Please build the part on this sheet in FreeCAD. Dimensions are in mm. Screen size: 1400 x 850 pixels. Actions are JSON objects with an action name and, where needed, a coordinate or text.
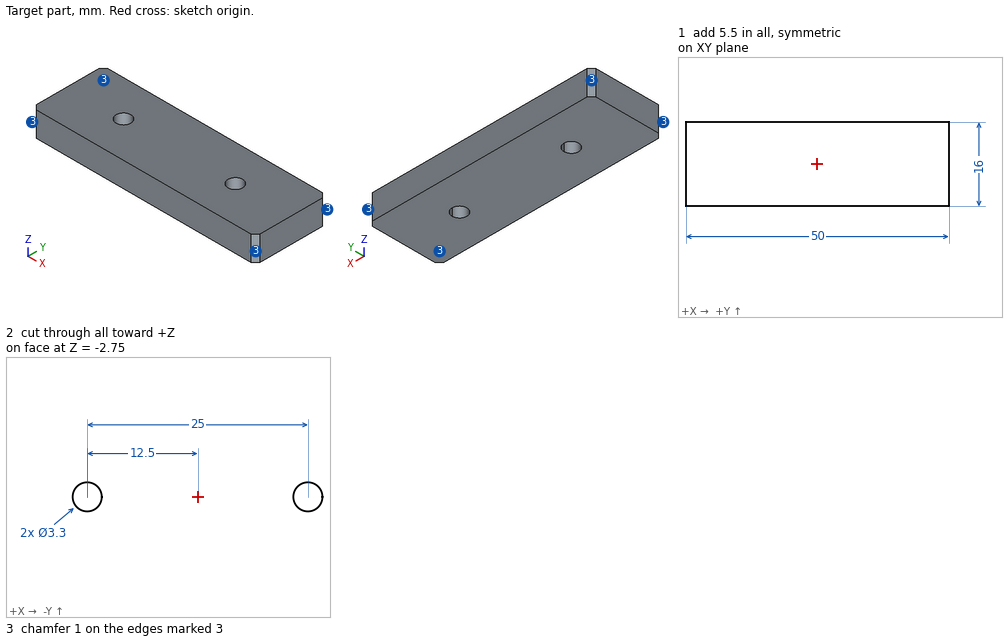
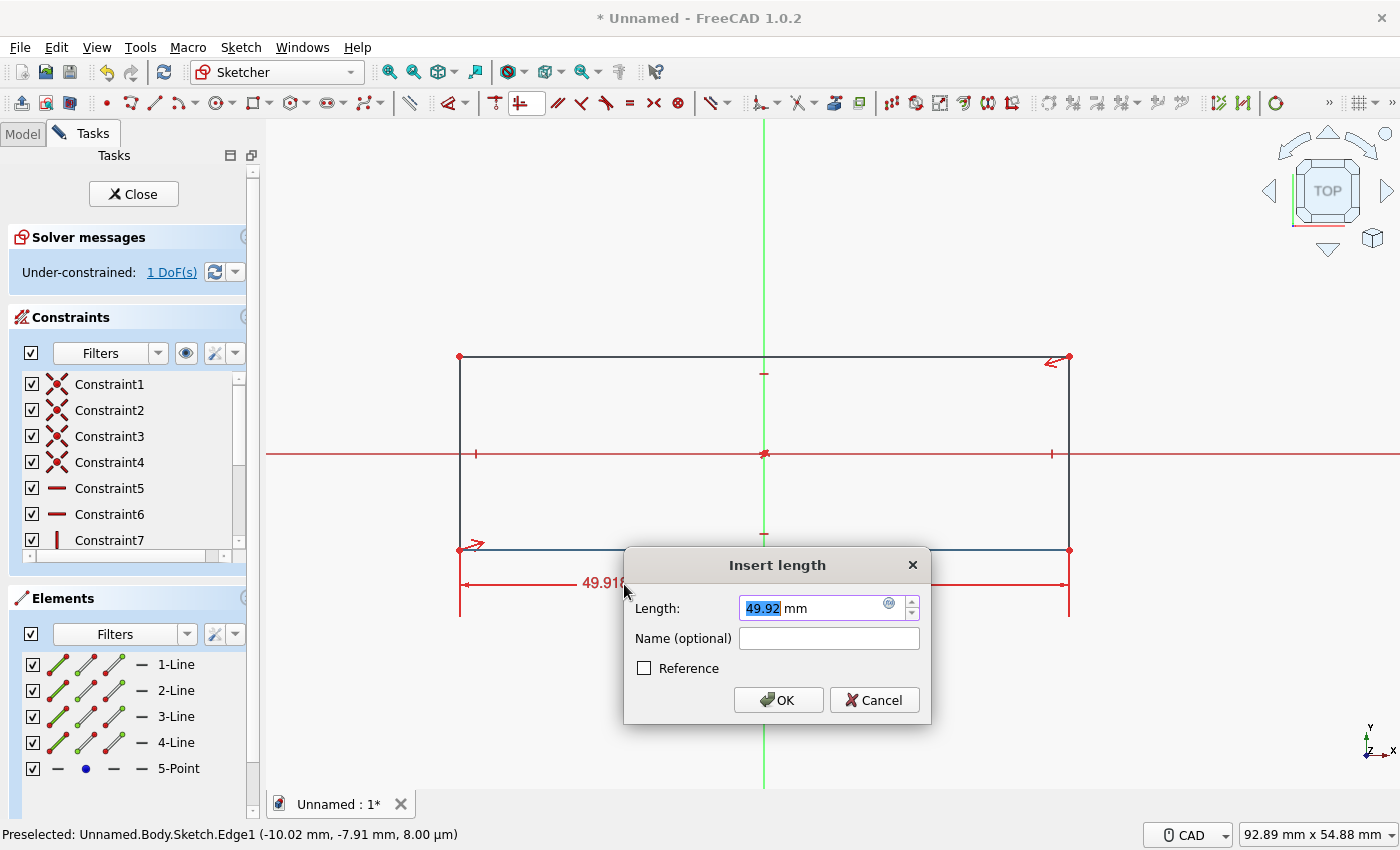
{"action": "type", "text": "50"}
{"action": "key", "text": "Return"}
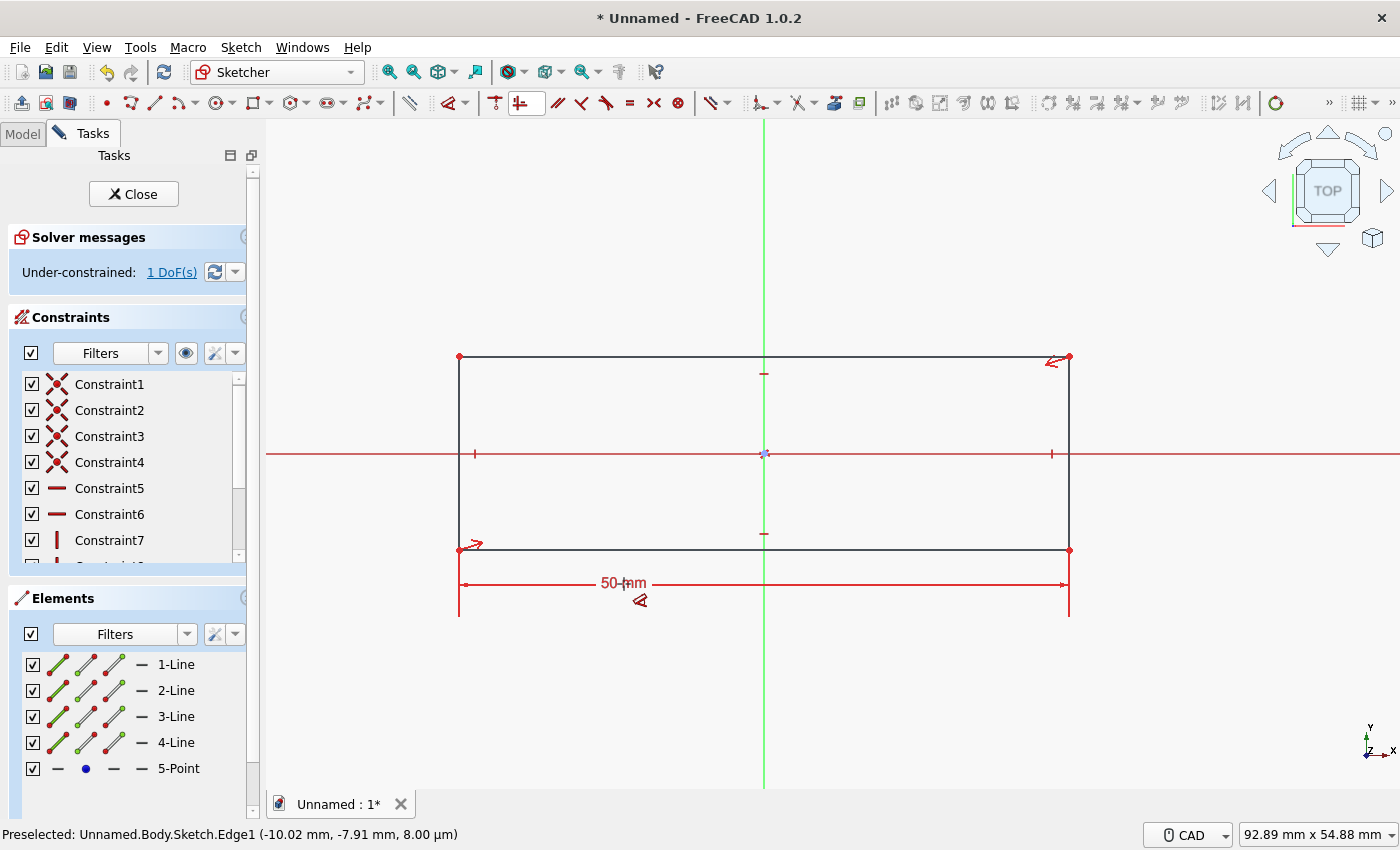
{"action": "left_click", "coordinate": [1069, 492]}
{"action": "left_click", "coordinate": [1103, 409]}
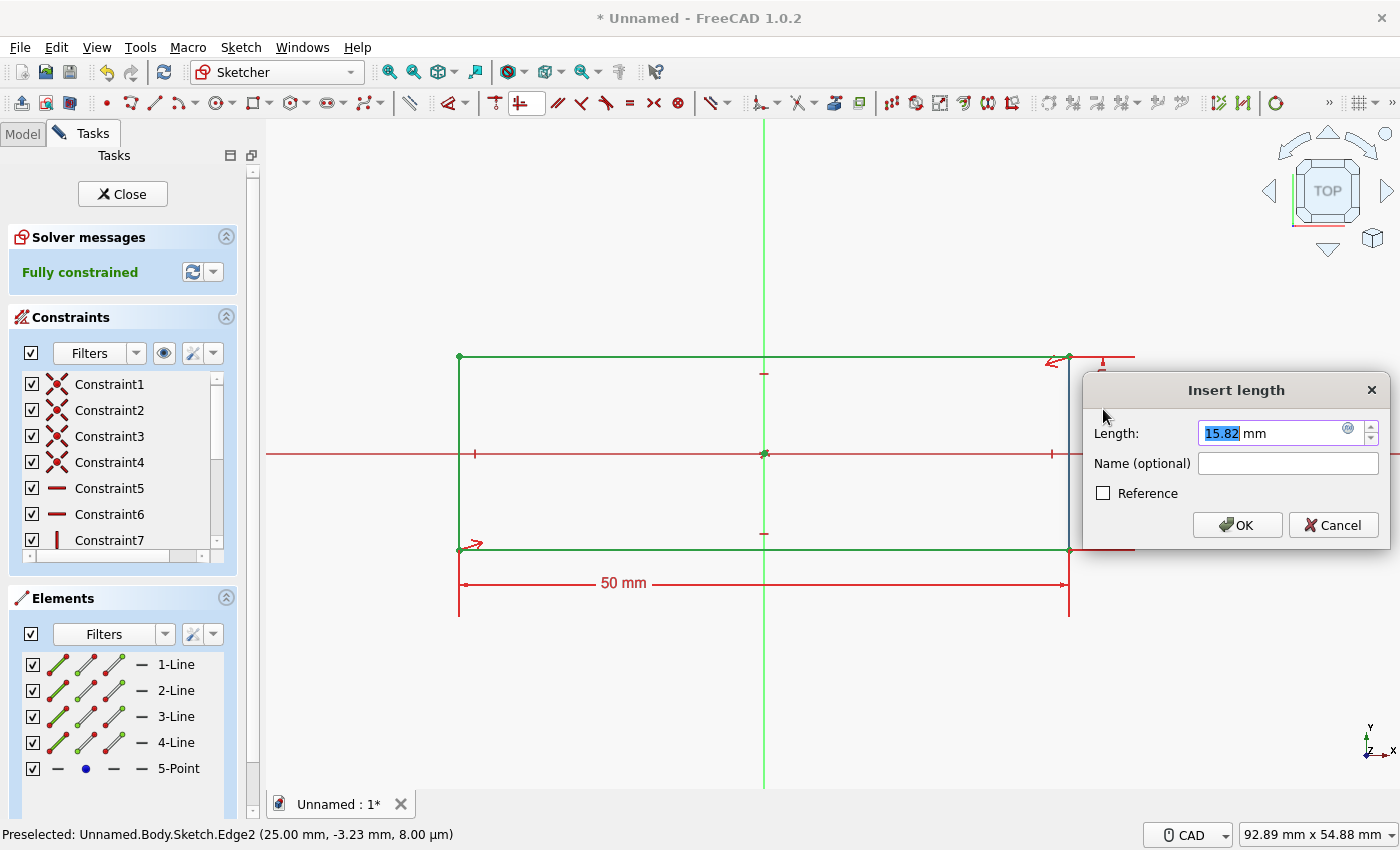
{"action": "type", "text": "16"}
{"action": "key", "text": "Return"}
{"action": "key", "text": "Escape"}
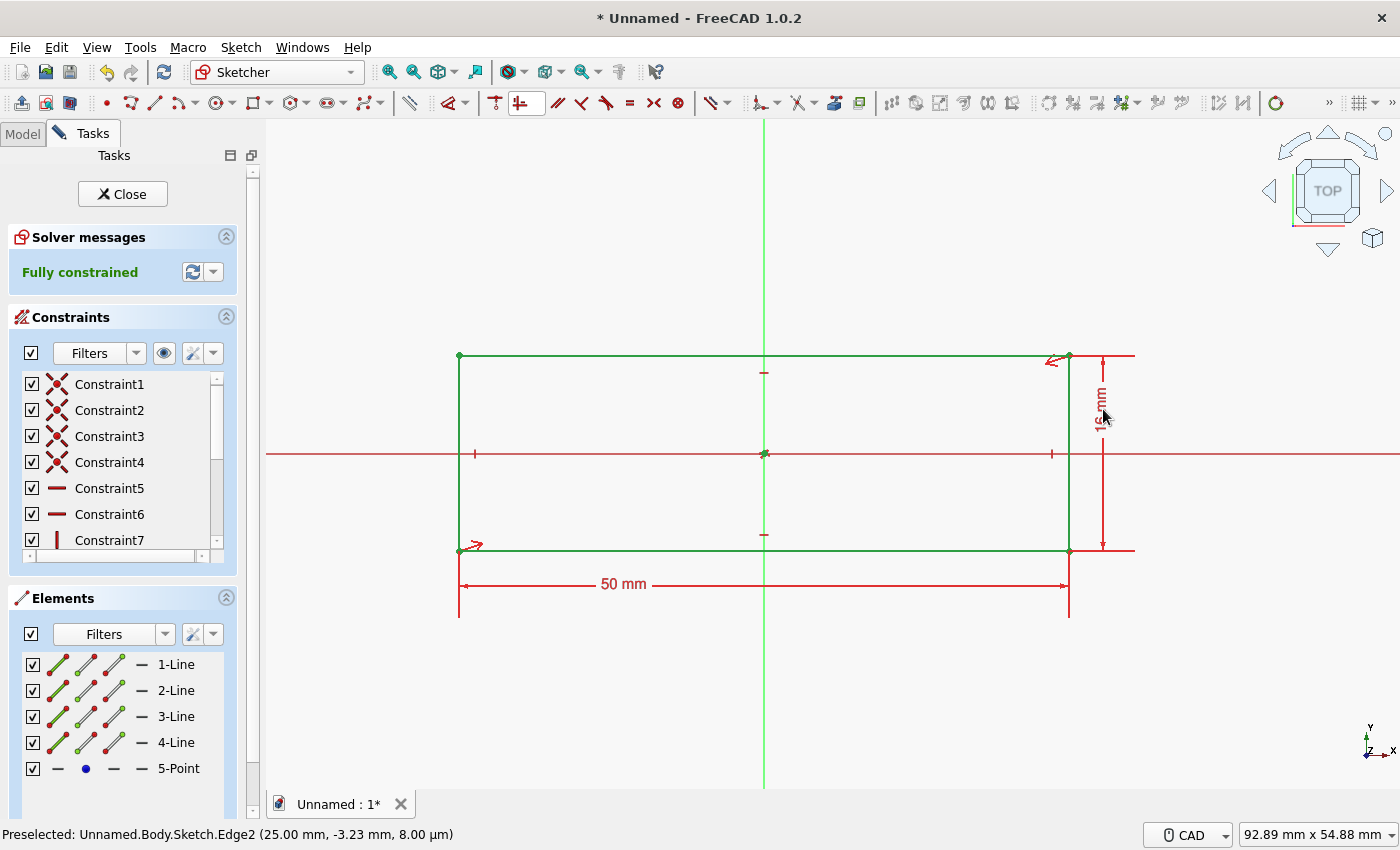
{"action": "left_click", "coordinate": [123, 194]}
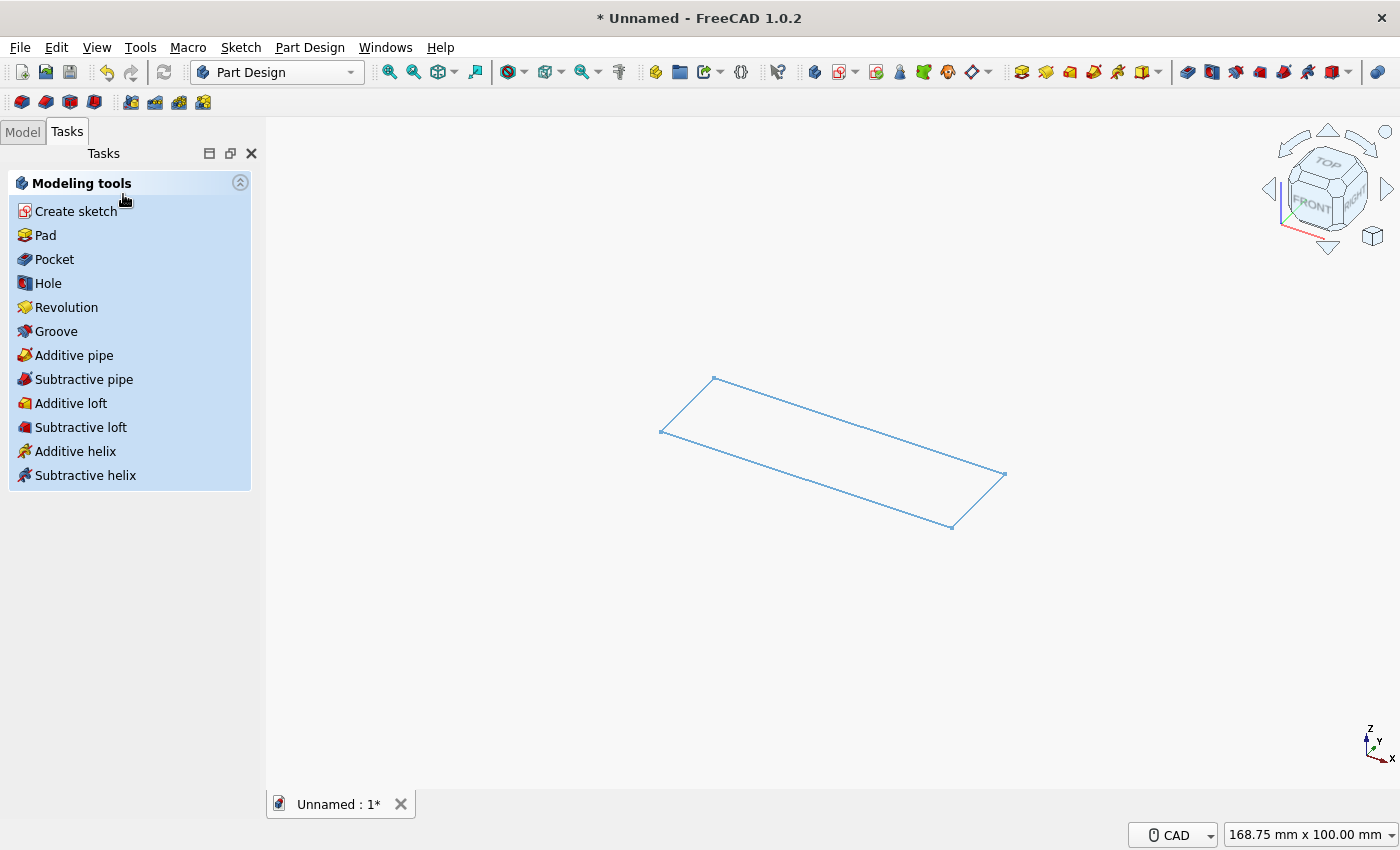
{"action": "left_click", "coordinate": [1022, 72]}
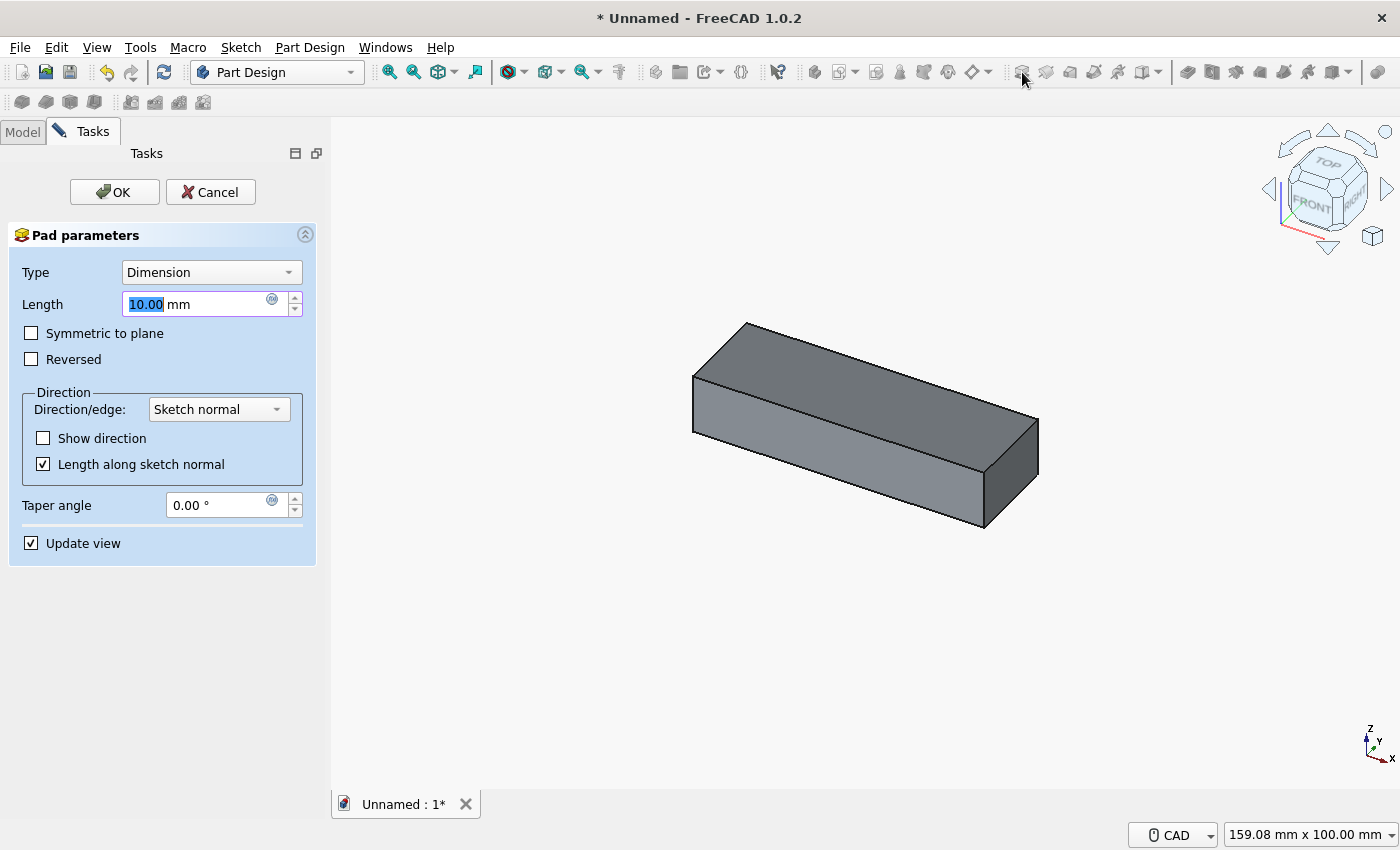
{"action": "type", "text": "5.5"}
{"action": "key", "text": "Tab"}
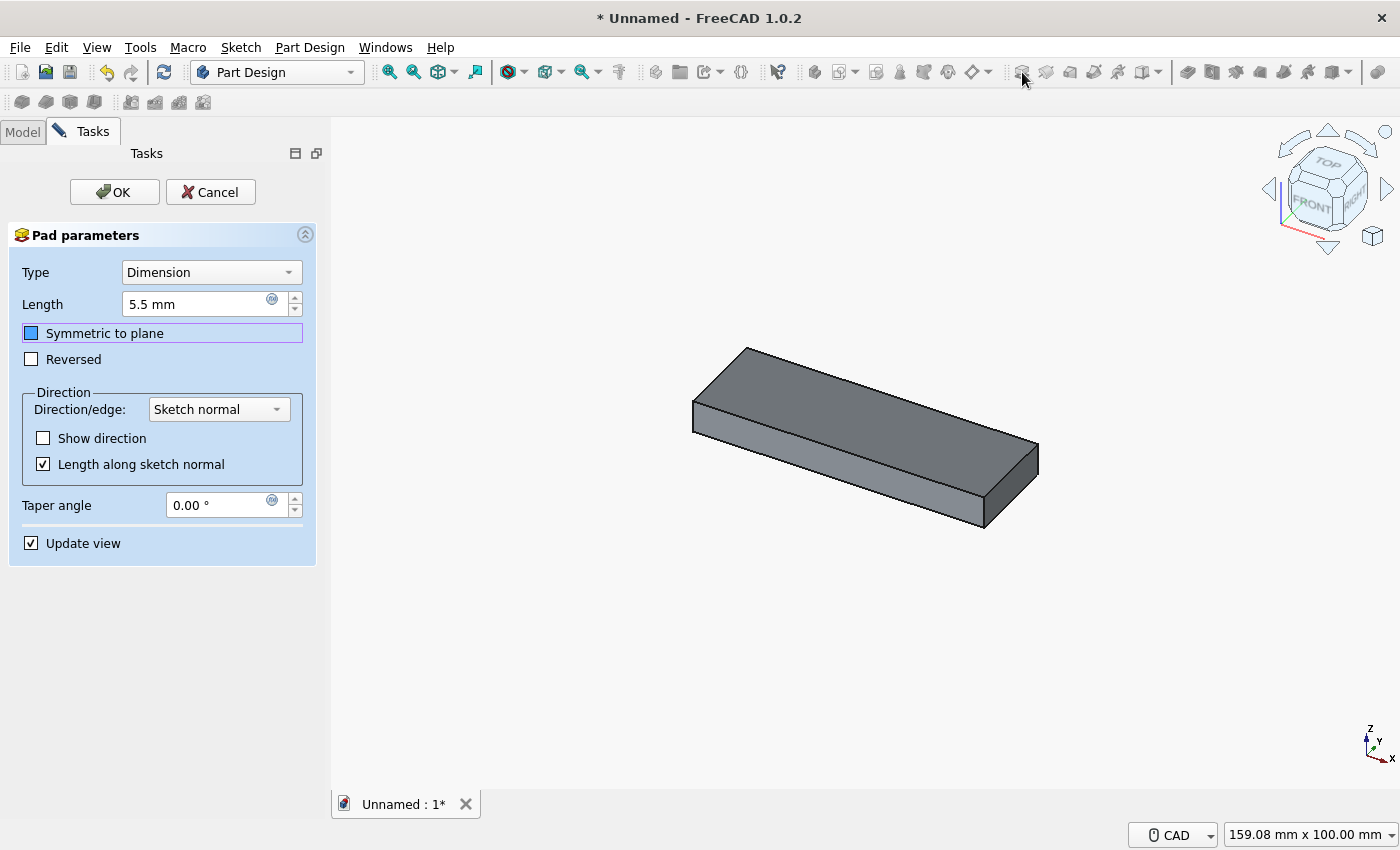
{"action": "left_click", "coordinate": [30, 333]}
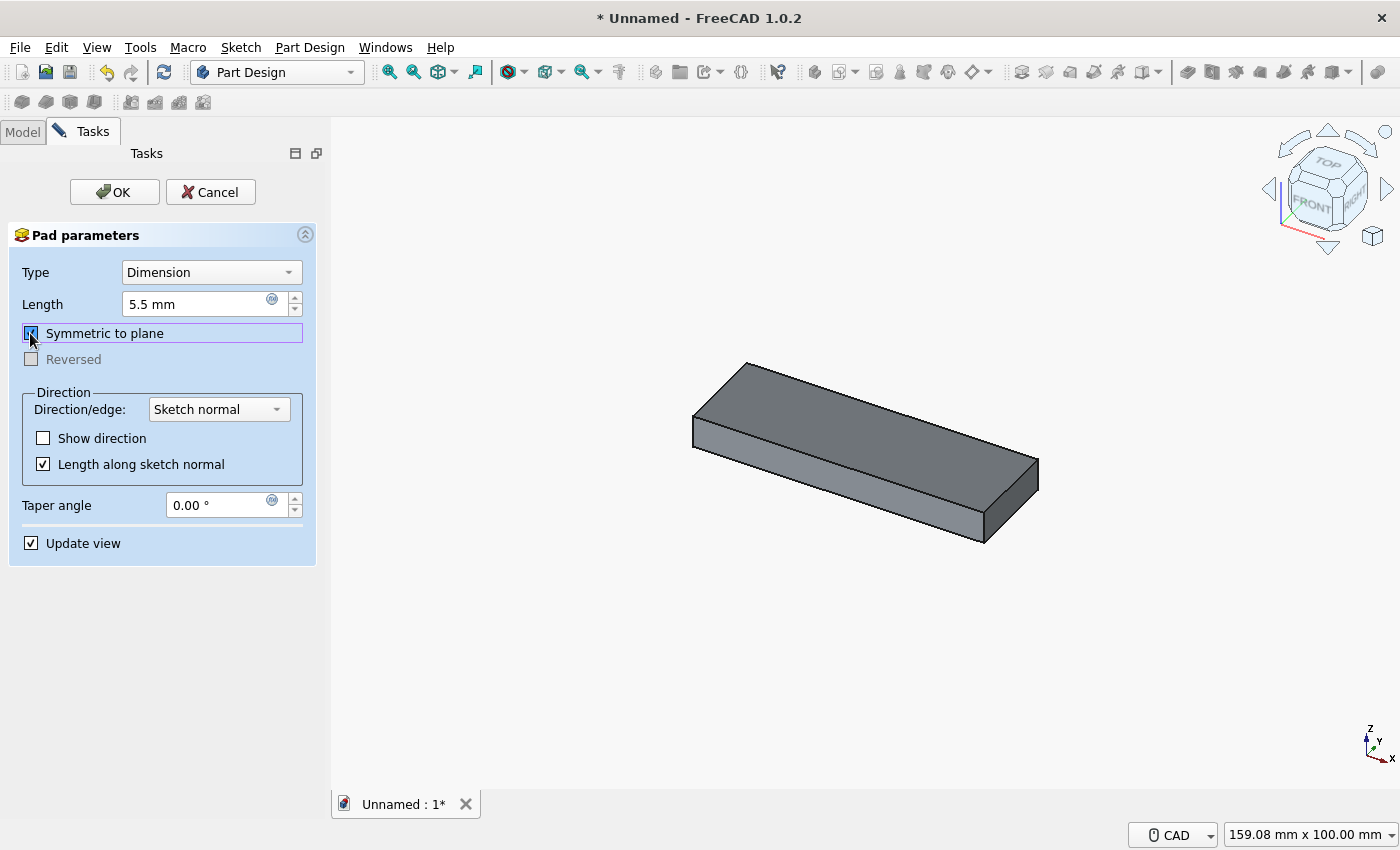
{"action": "left_click", "coordinate": [115, 192]}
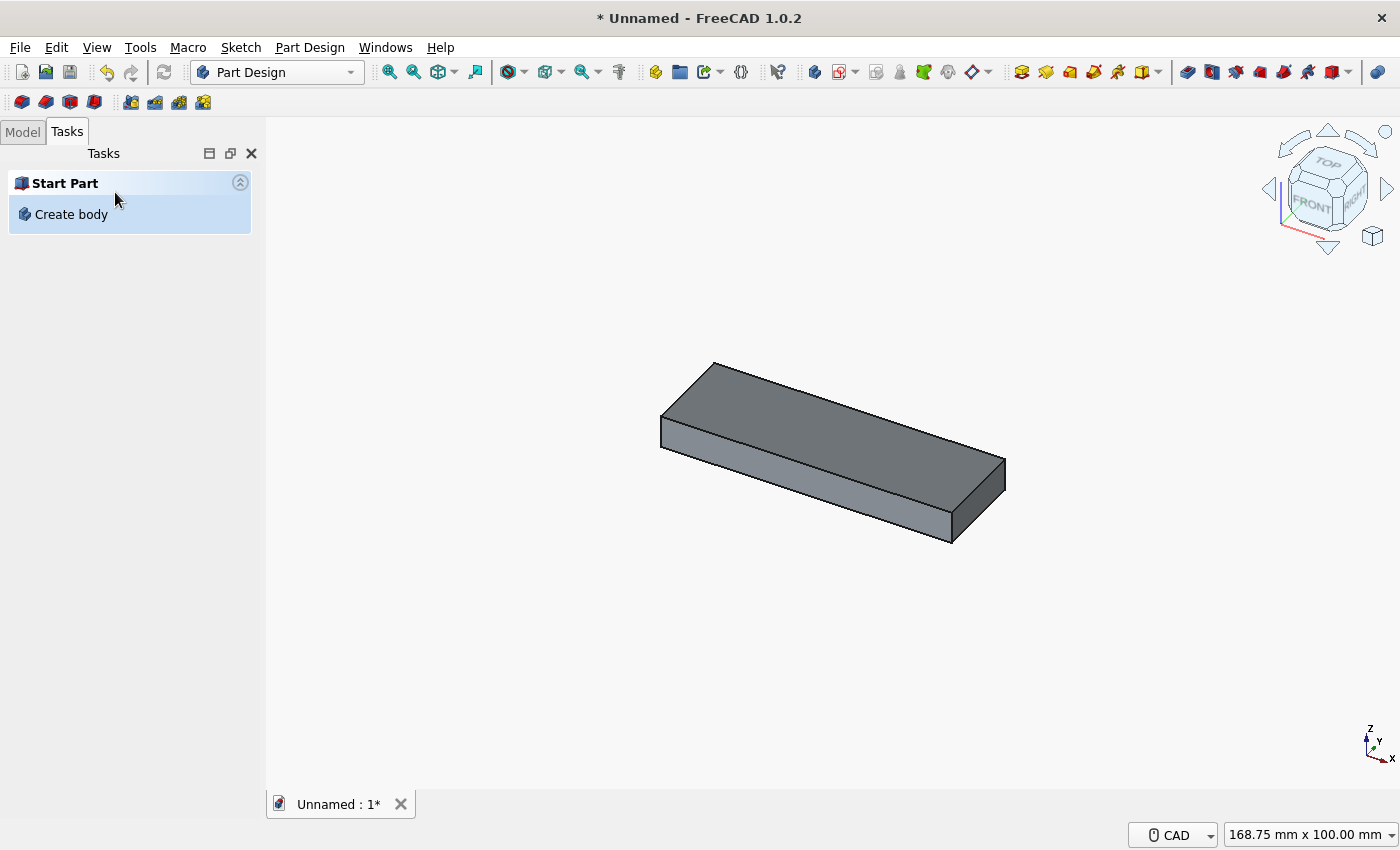
{"action": "left_click", "coordinate": [390, 72]}